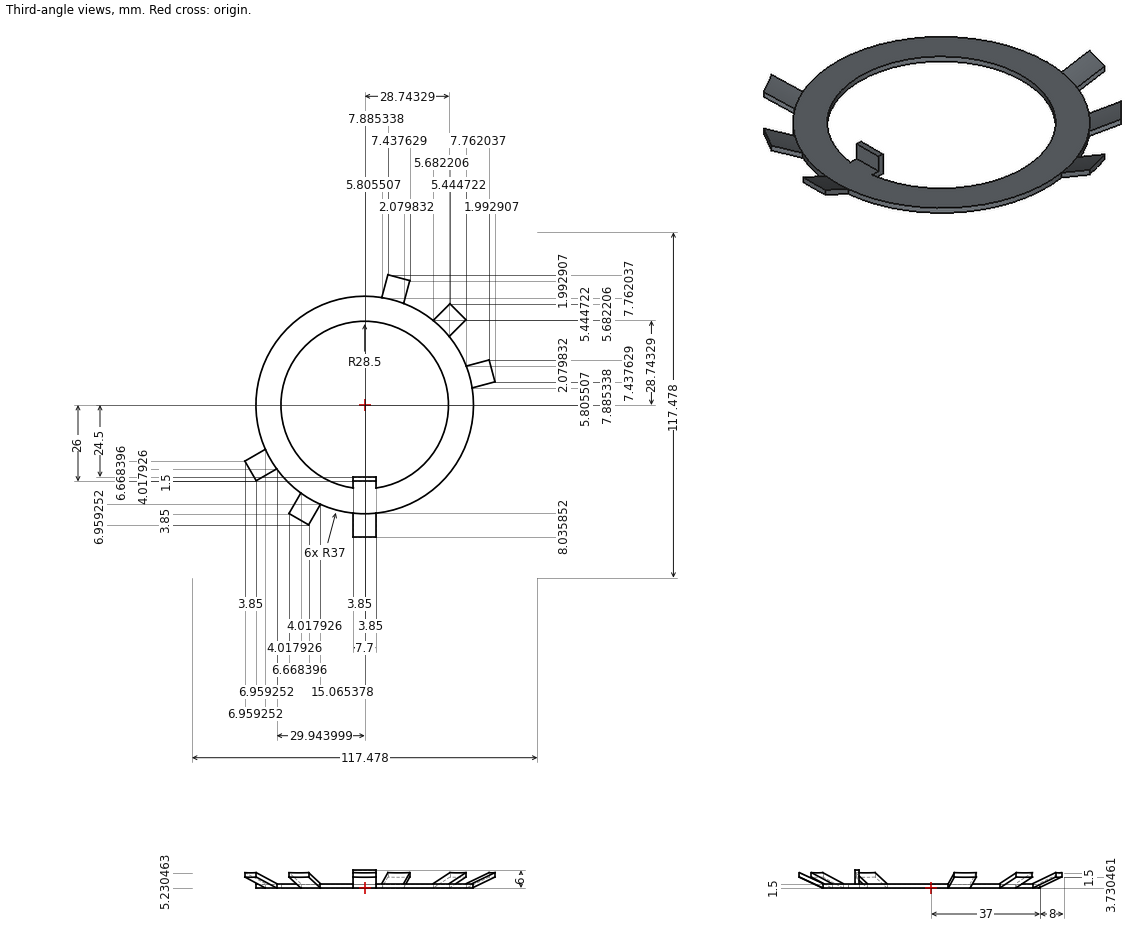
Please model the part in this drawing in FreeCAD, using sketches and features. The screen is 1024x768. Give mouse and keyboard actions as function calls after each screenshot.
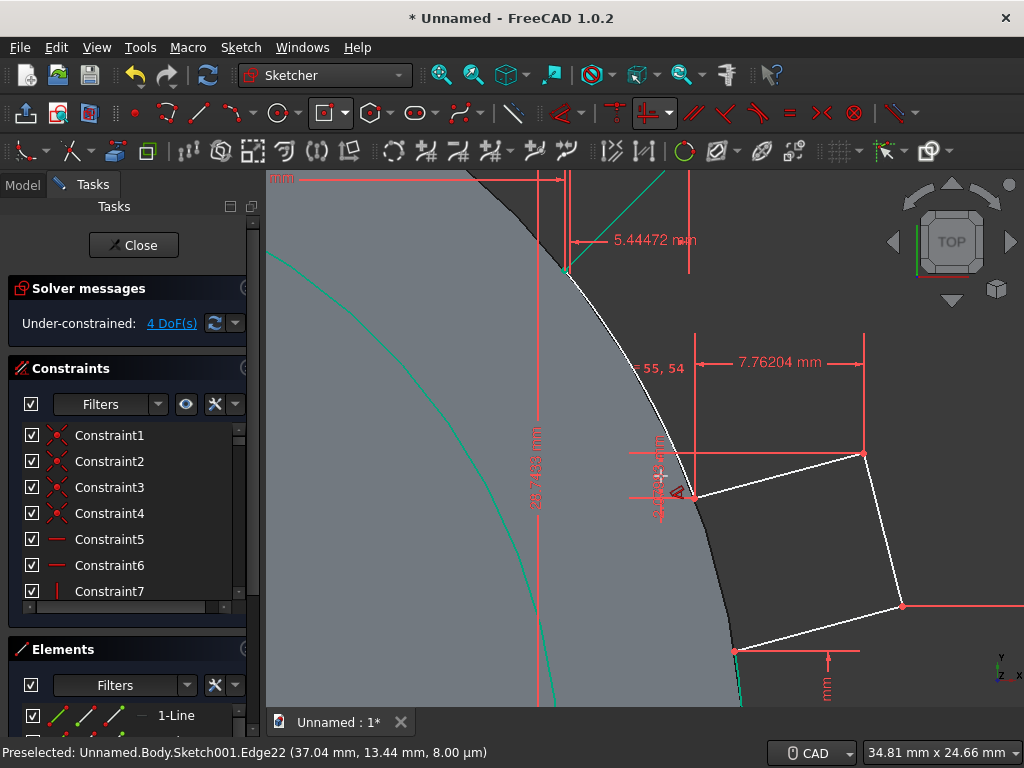
scroll(676, 385, down, 10)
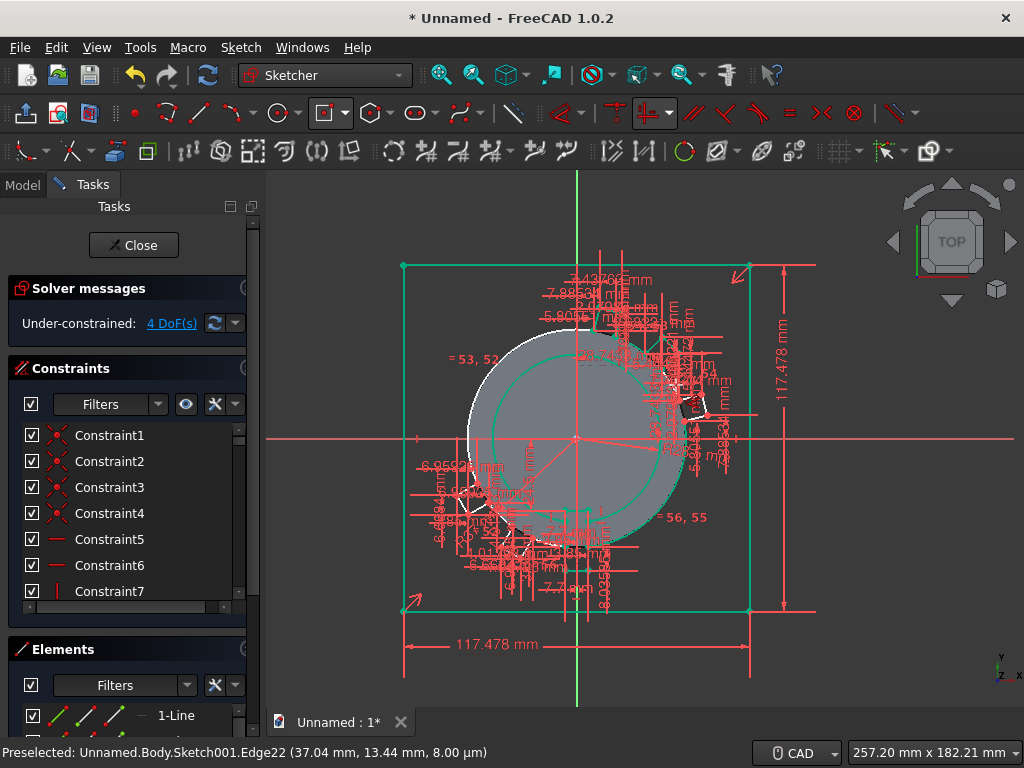
scroll(703, 401, up, 10)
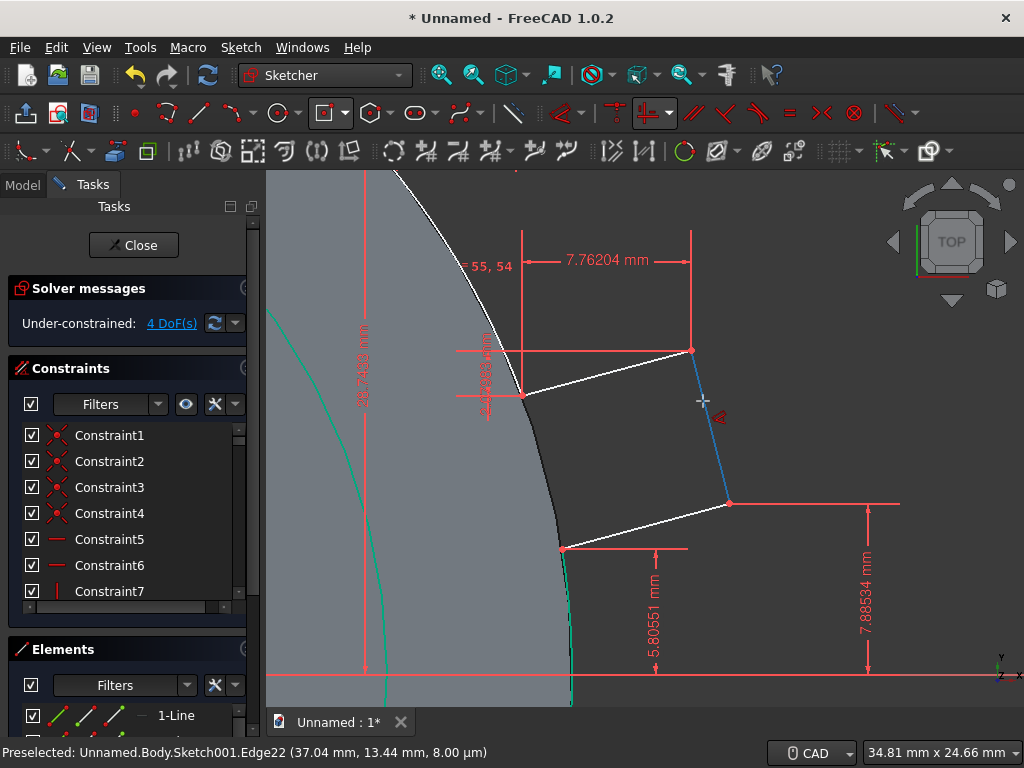
click(703, 397)
click(711, 317)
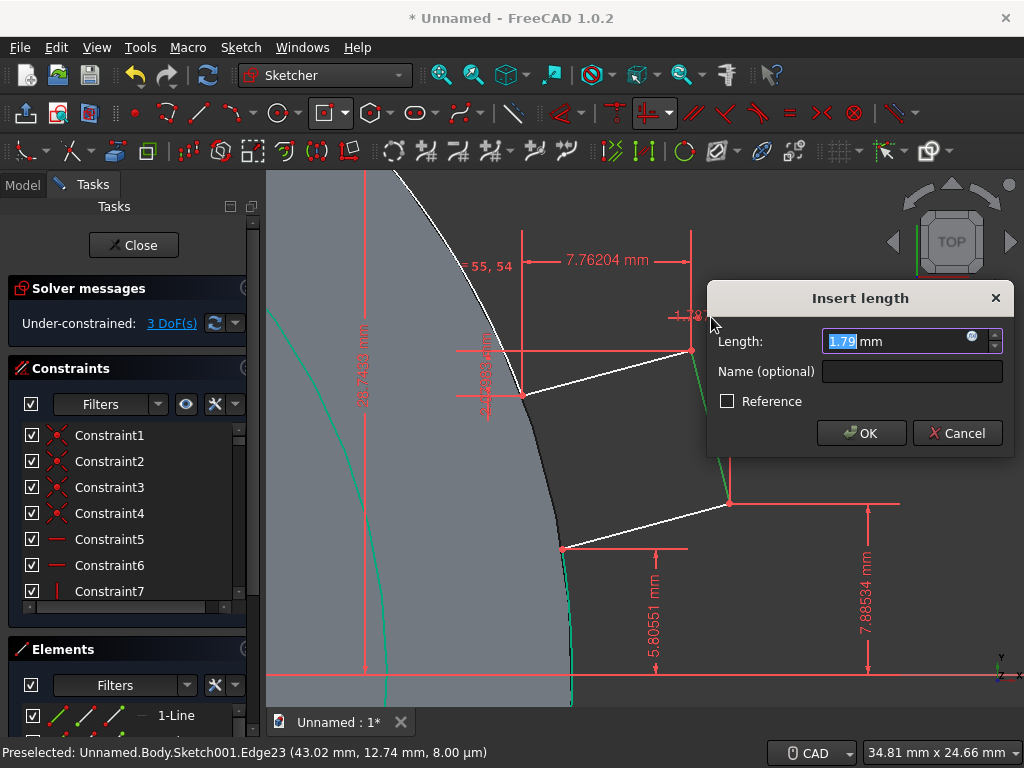
text(1.992907)
key(Return)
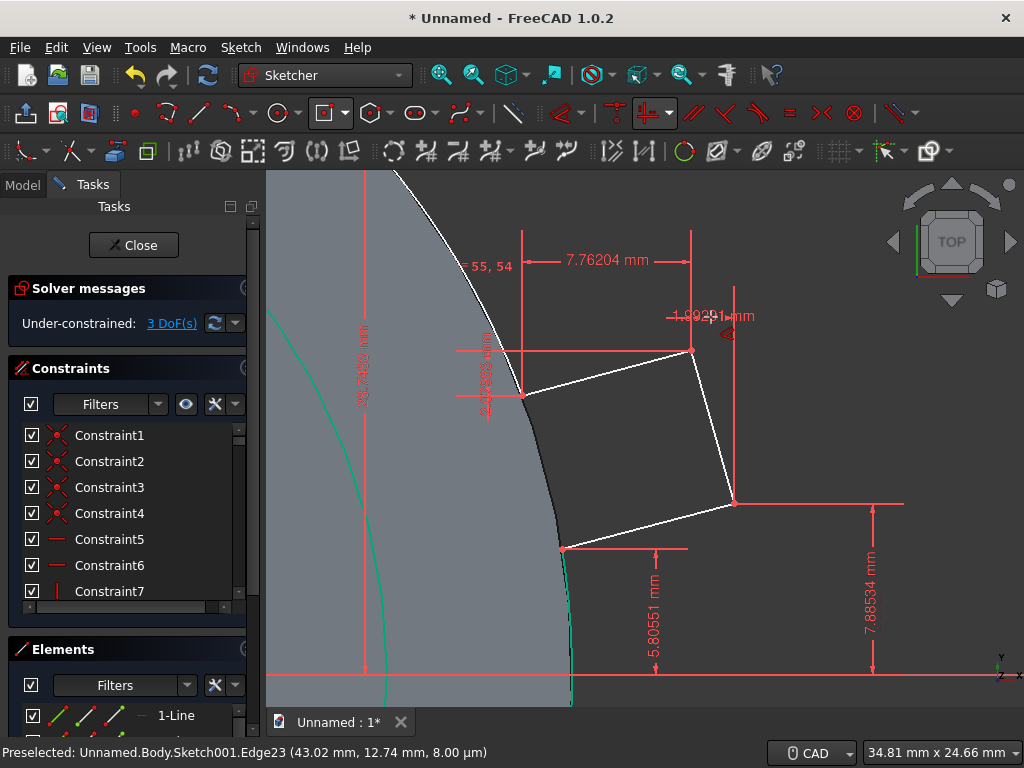
scroll(703, 401, down, 10)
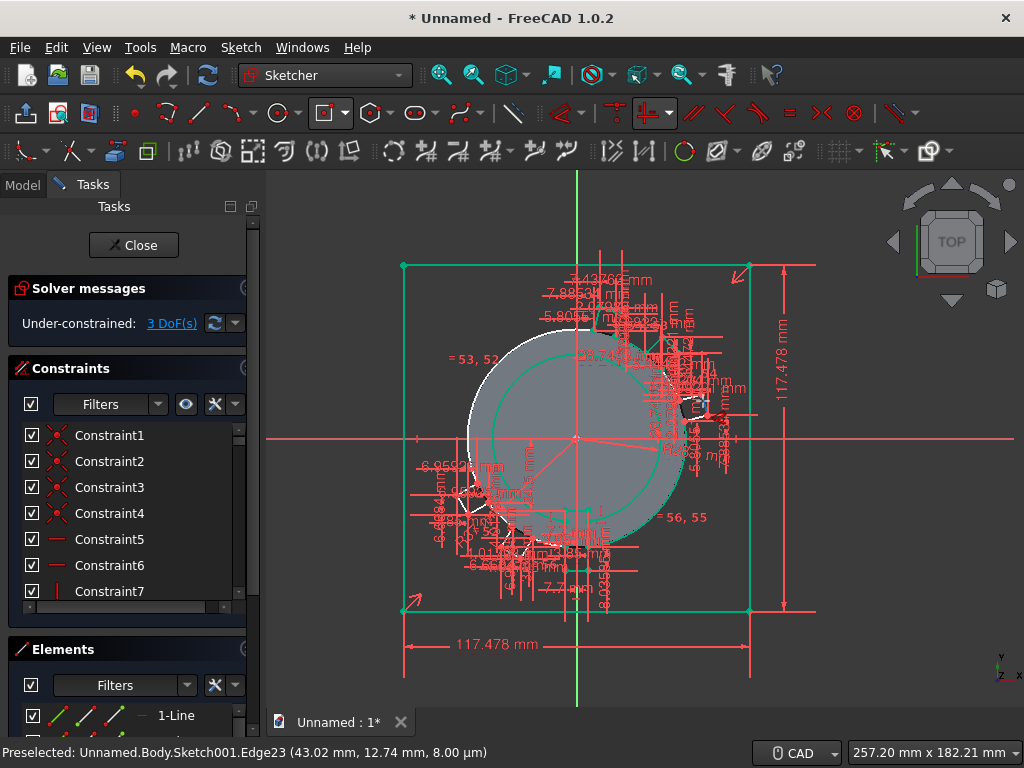
scroll(704, 401, up, 4)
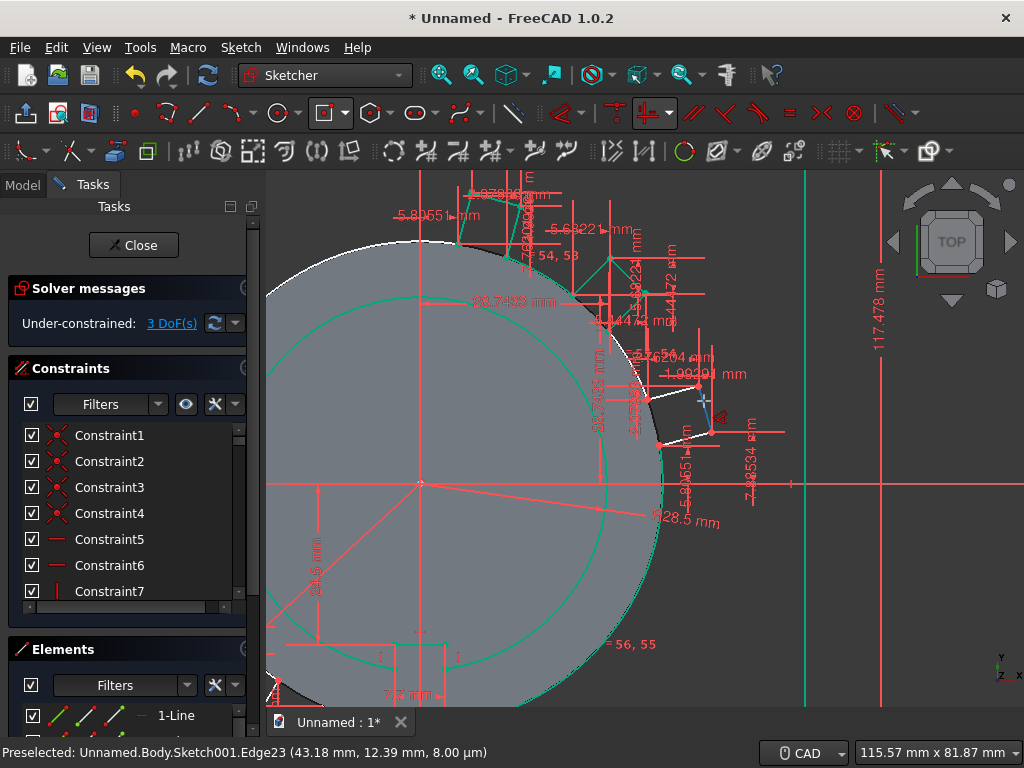
click(703, 400)
click(746, 409)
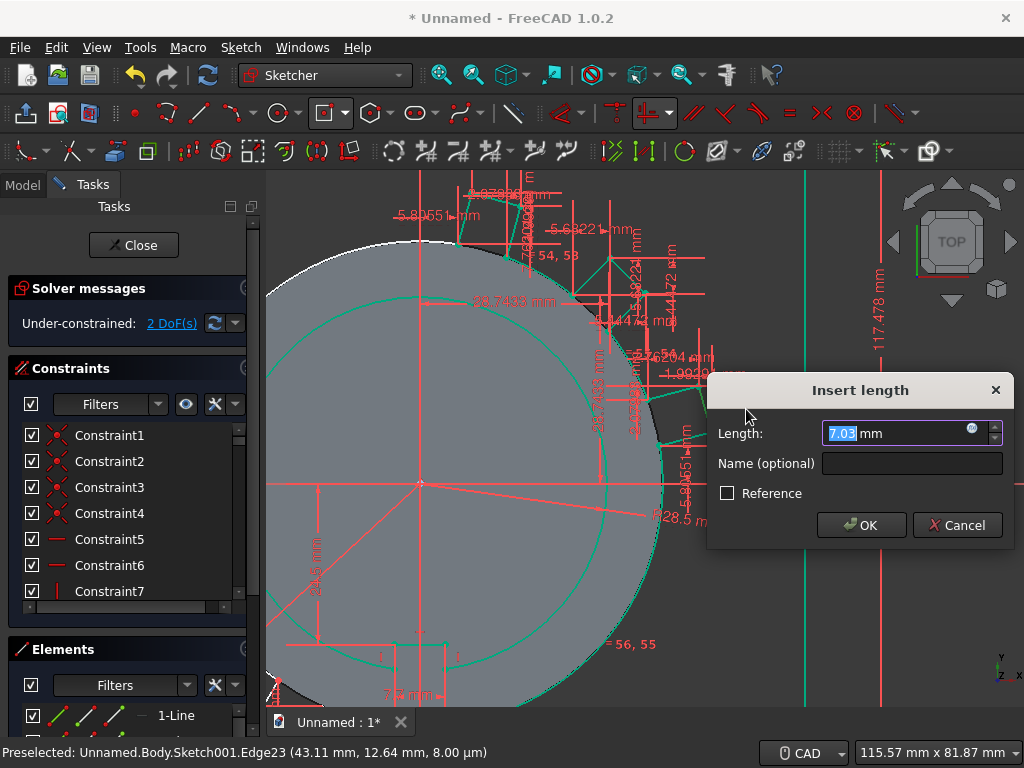
text(7.437629)
key(Return)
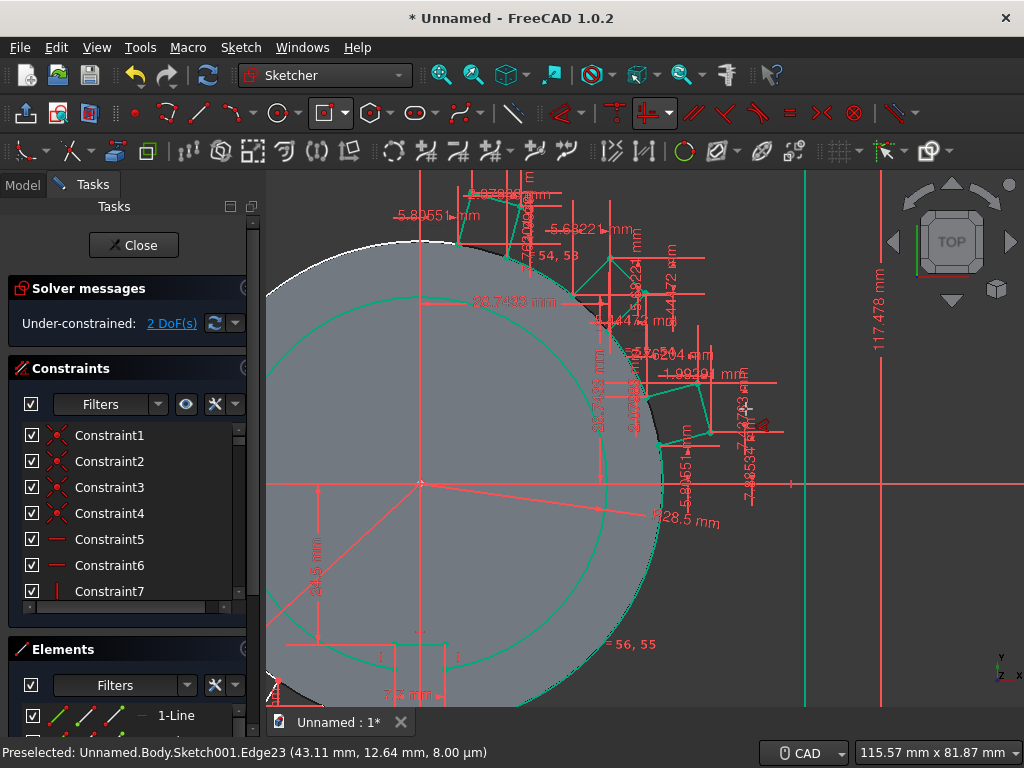
scroll(704, 401, down, 4)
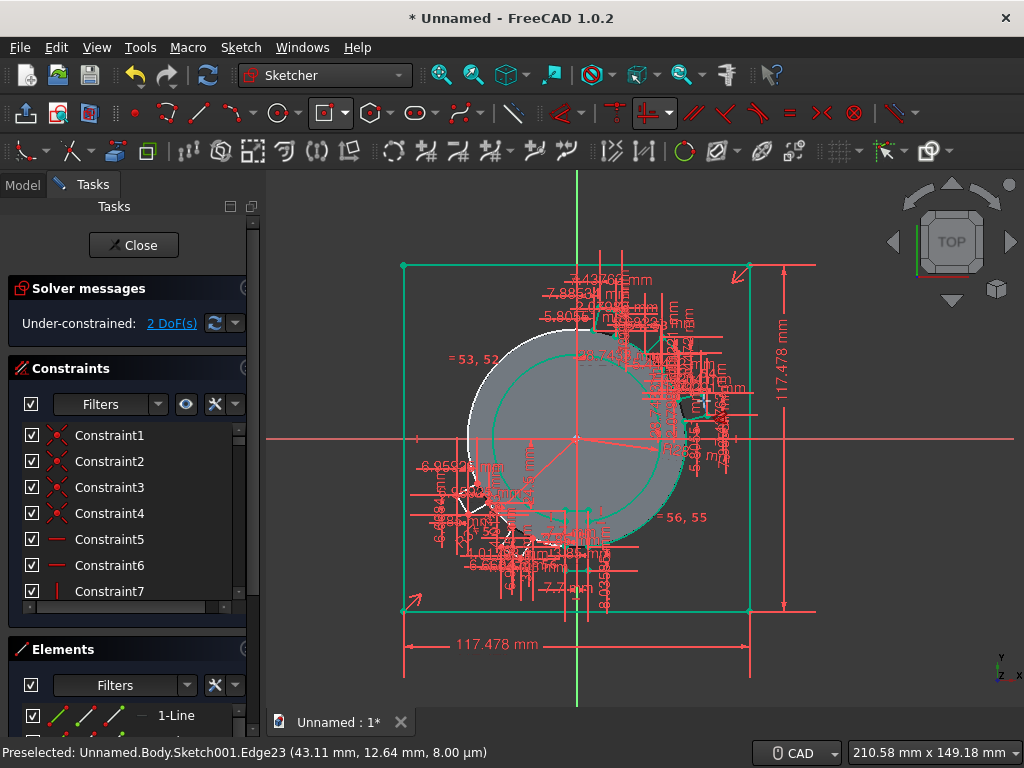
click(533, 538)
click(555, 405)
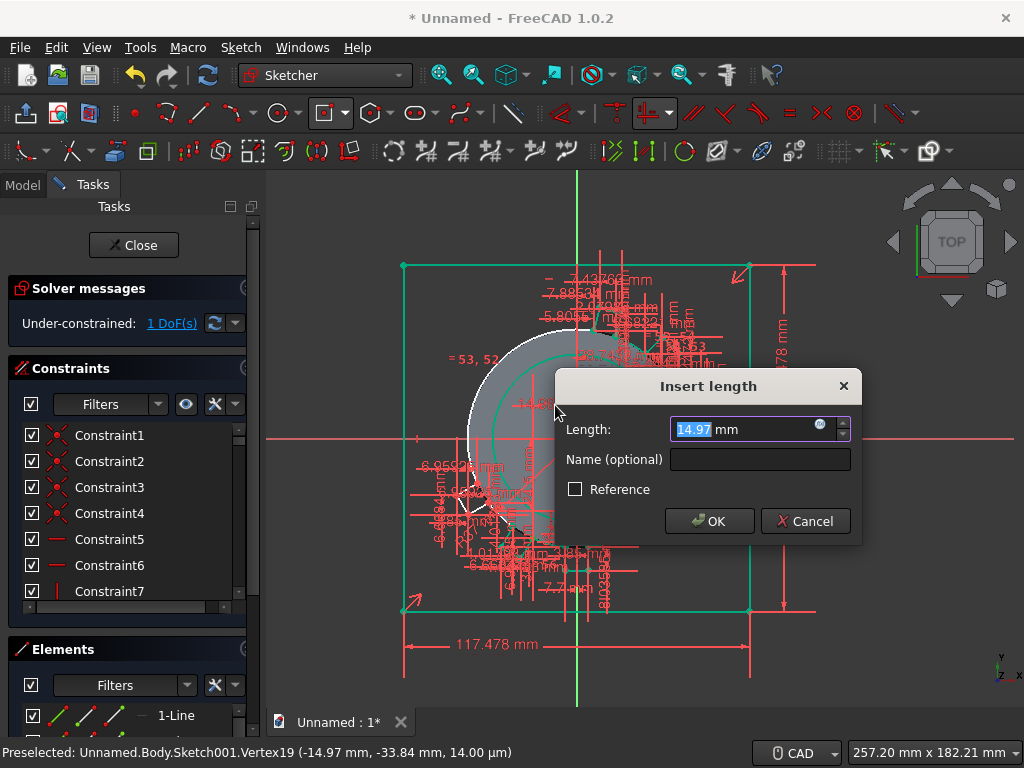
text(15.065378)
key(Return)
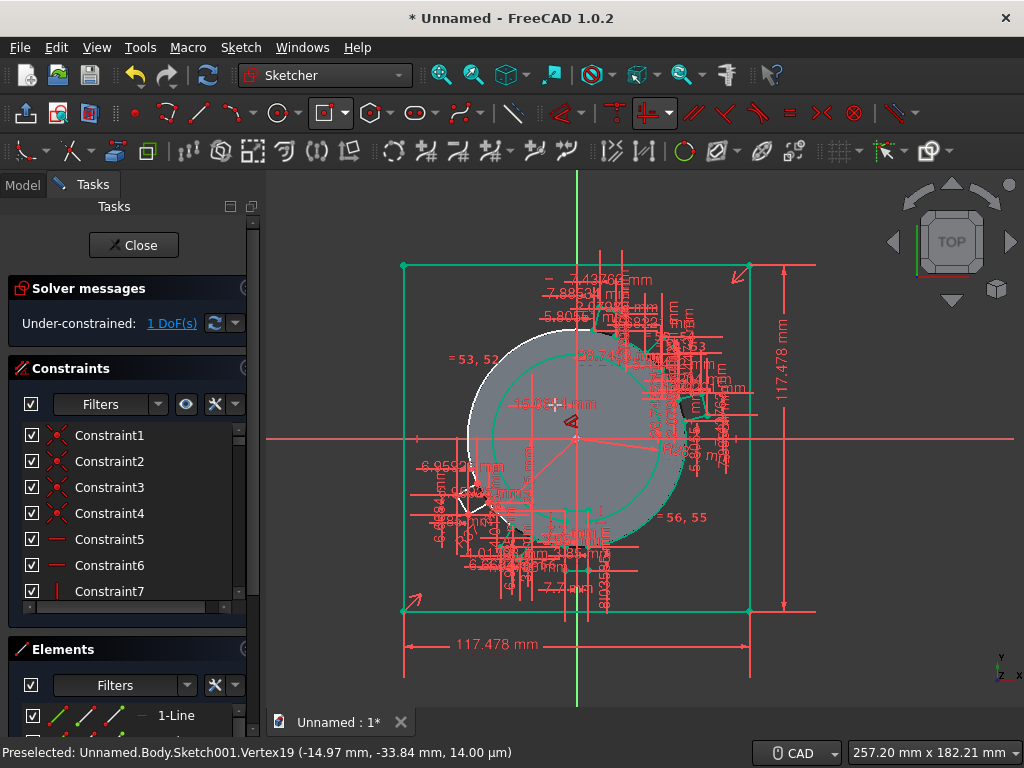
click(489, 503)
click(553, 381)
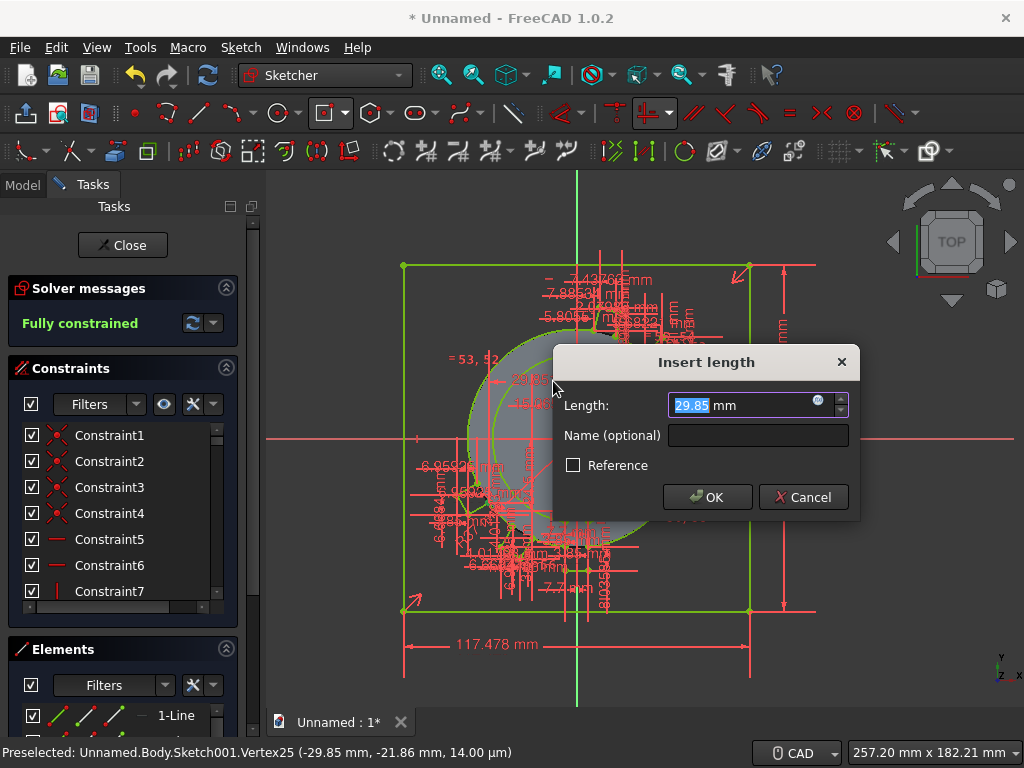
text(29.943999)
key(Return)
key(Escape)